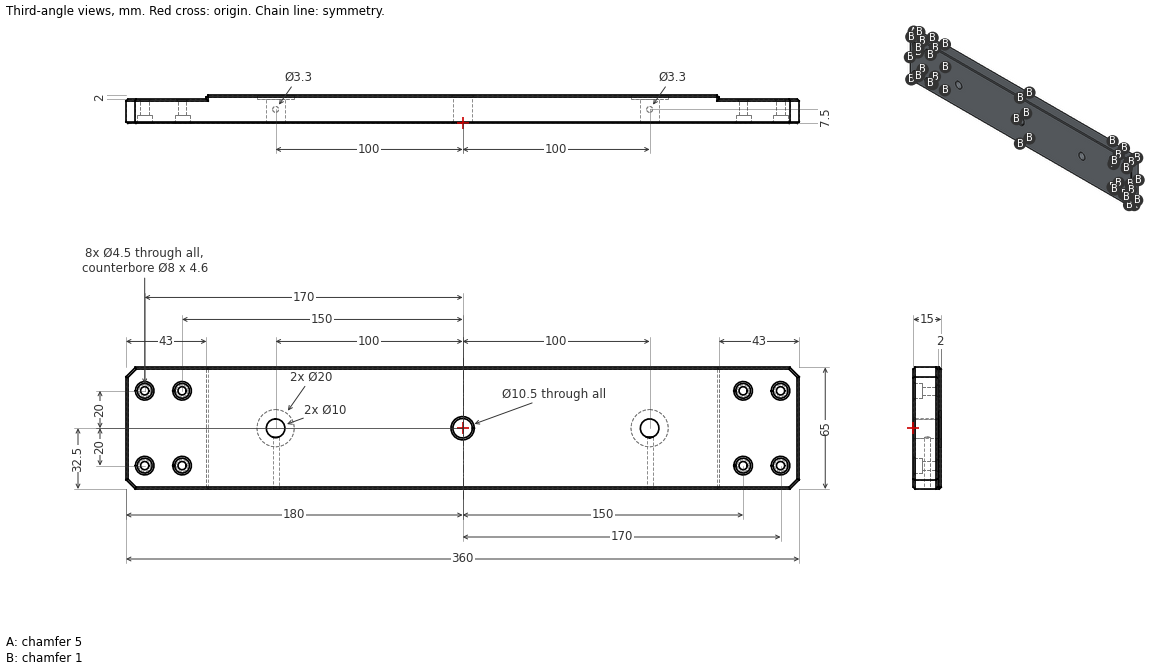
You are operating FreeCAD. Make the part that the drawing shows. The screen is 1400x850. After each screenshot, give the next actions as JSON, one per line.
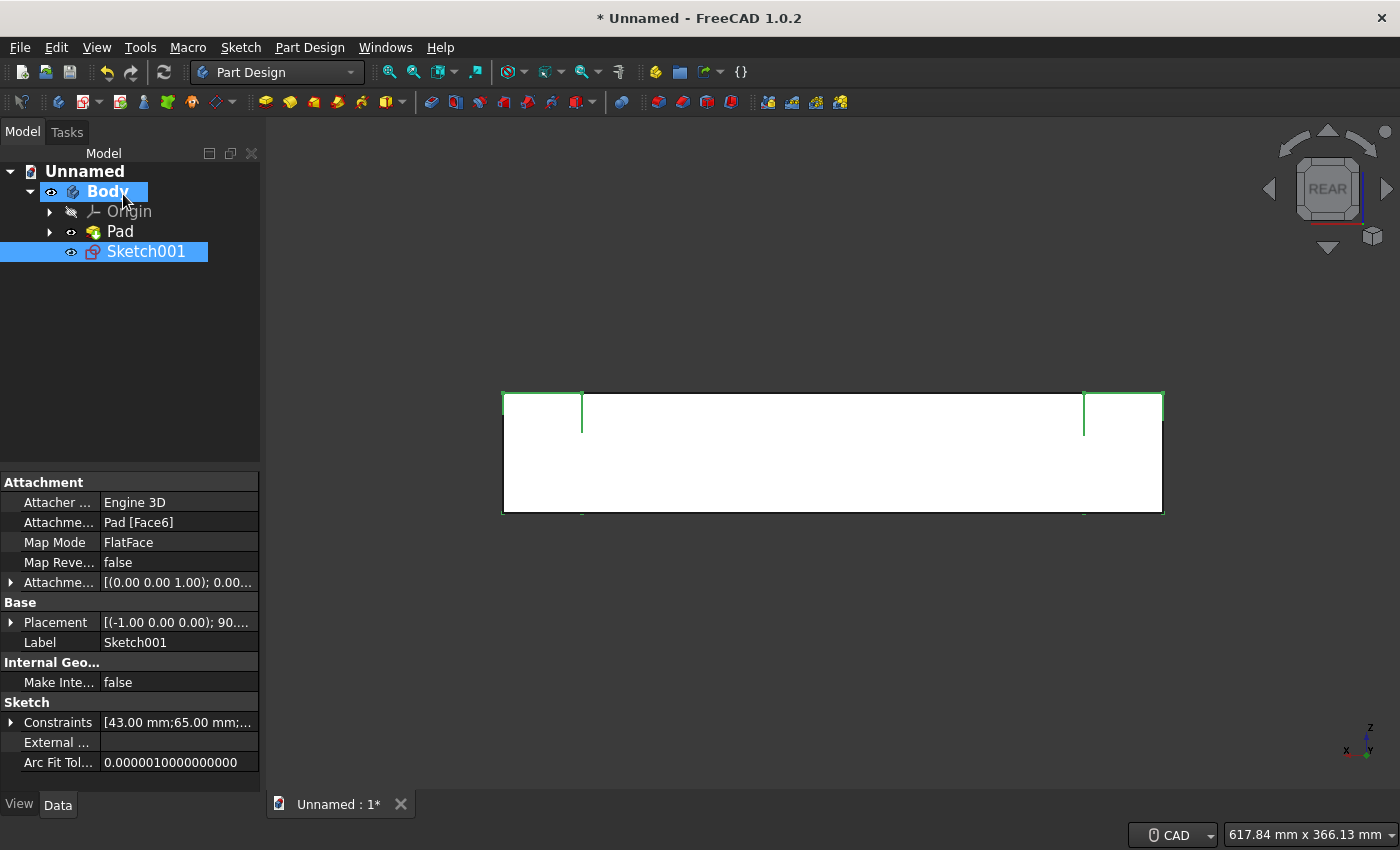
{"action": "left_click", "coordinate": [432, 102]}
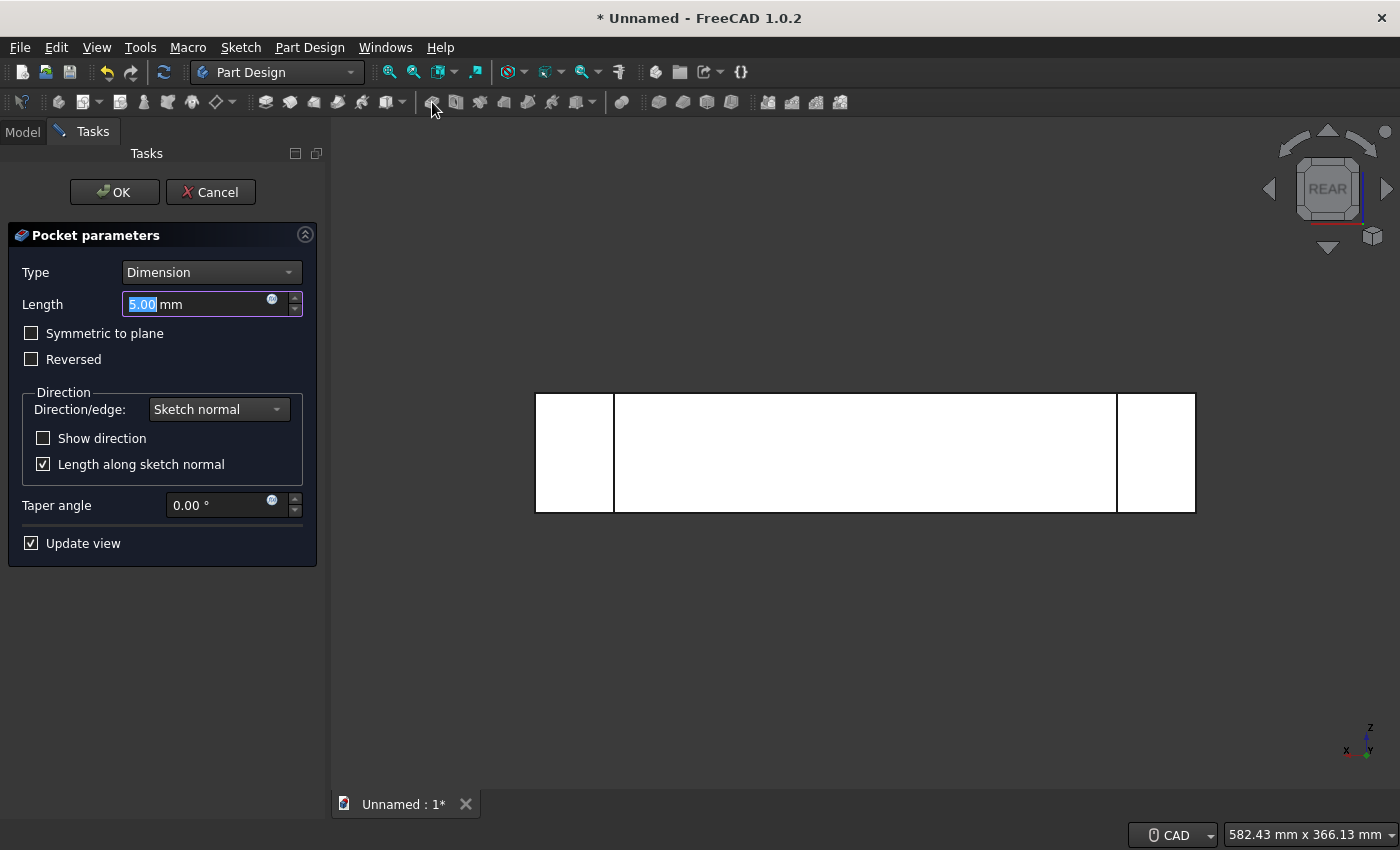
{"action": "type", "text": "2"}
{"action": "key", "text": "Tab"}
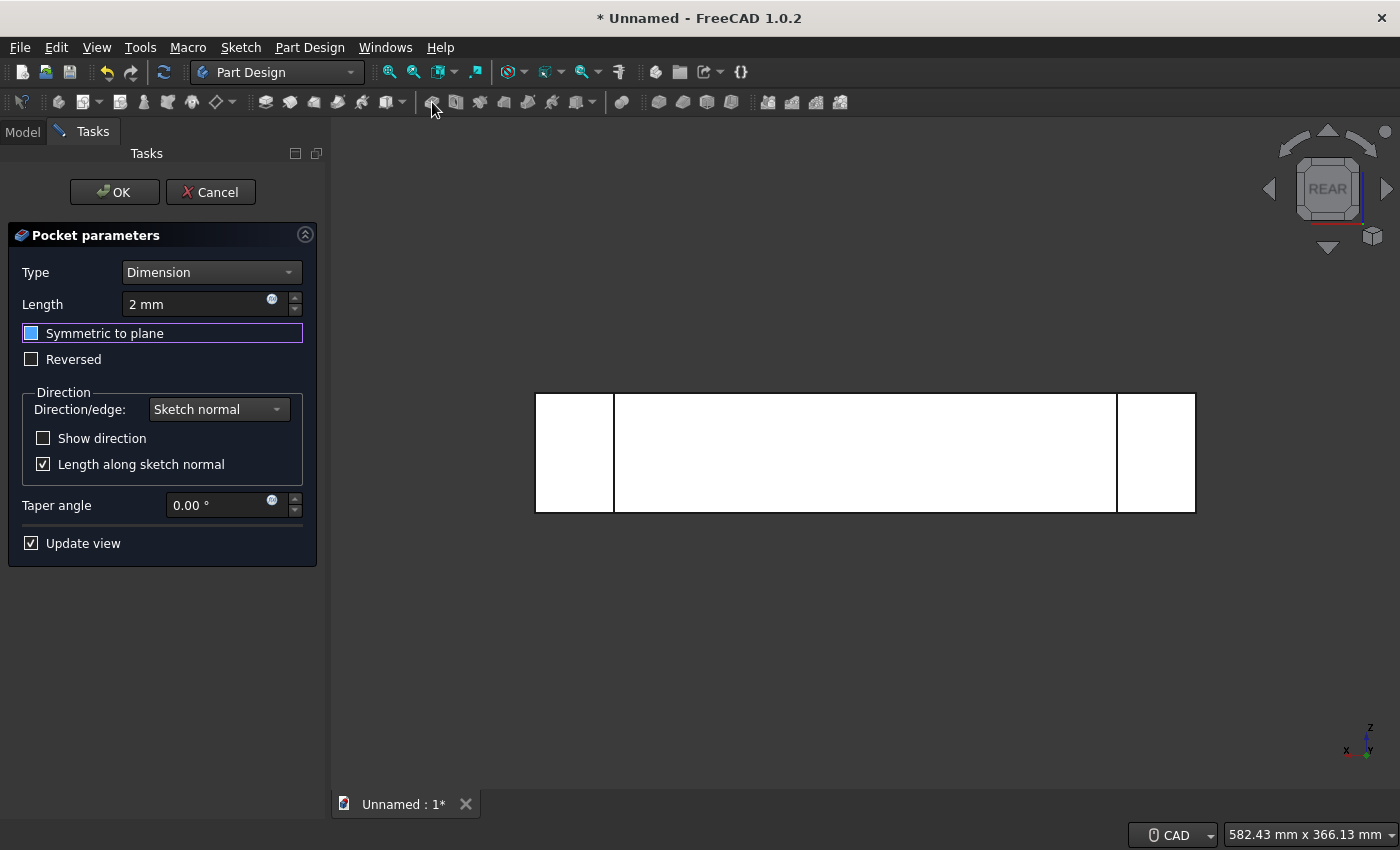
{"action": "left_click", "coordinate": [115, 192]}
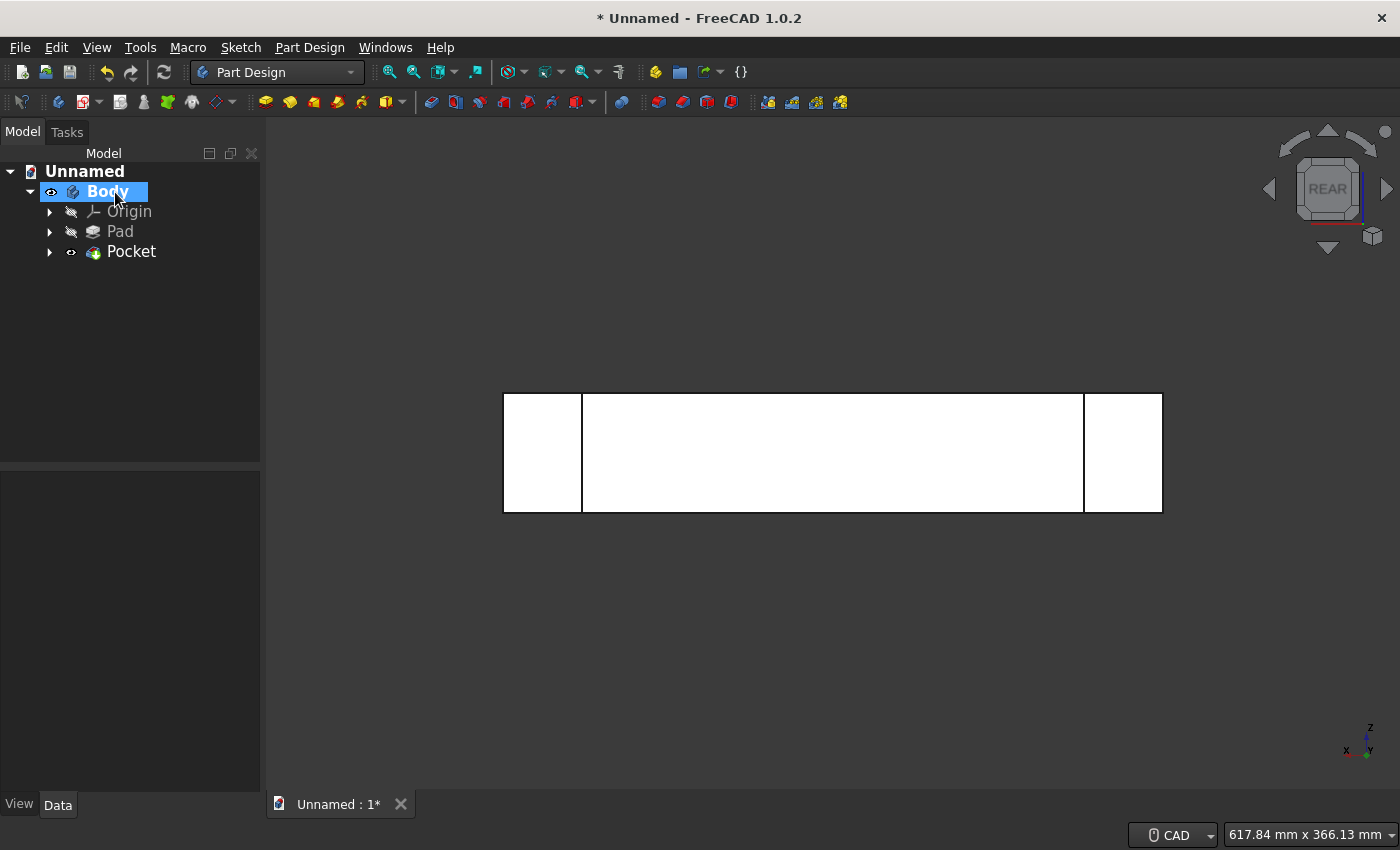
{"action": "left_click", "coordinate": [84, 102]}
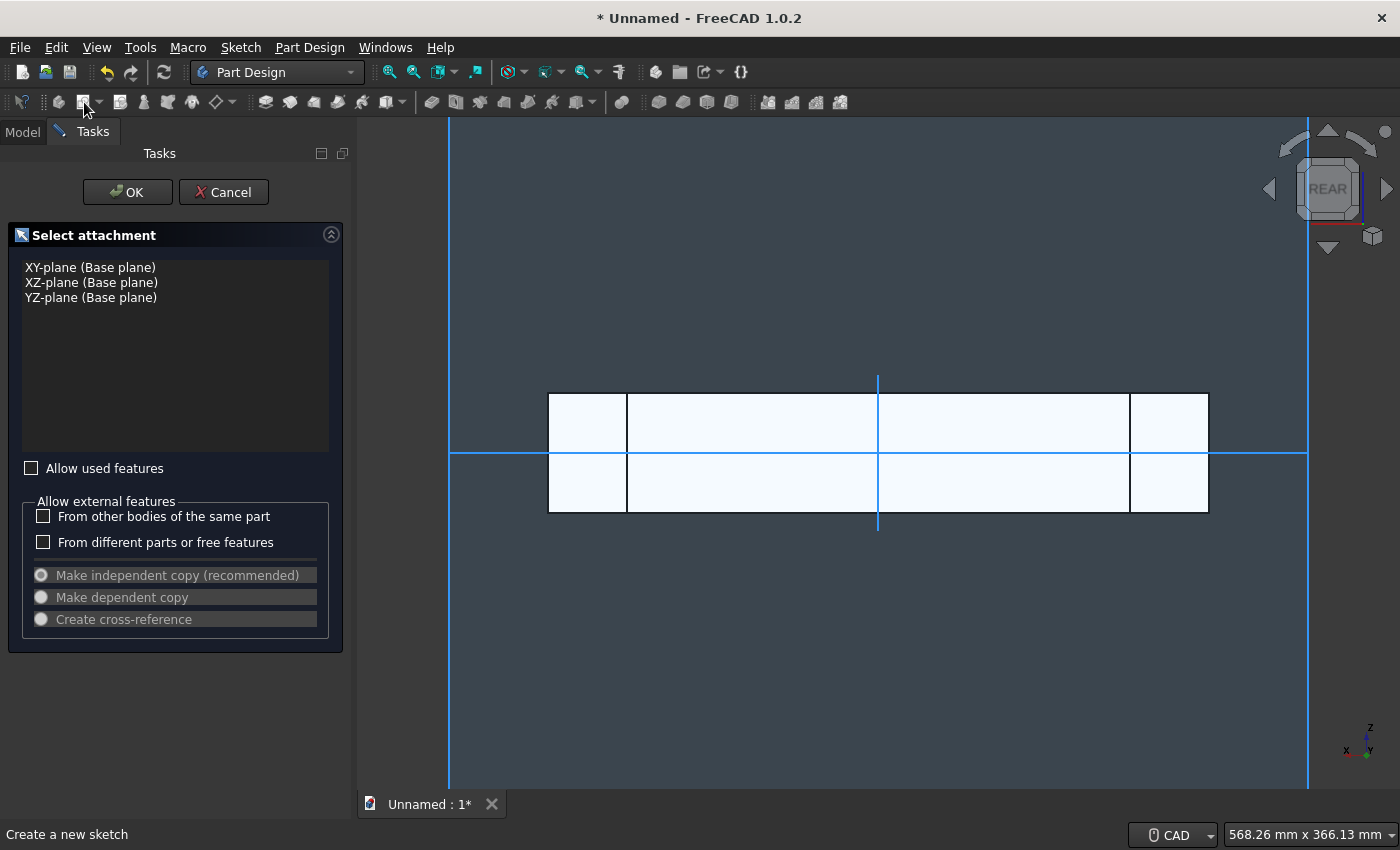
{"action": "left_click", "coordinate": [82, 282]}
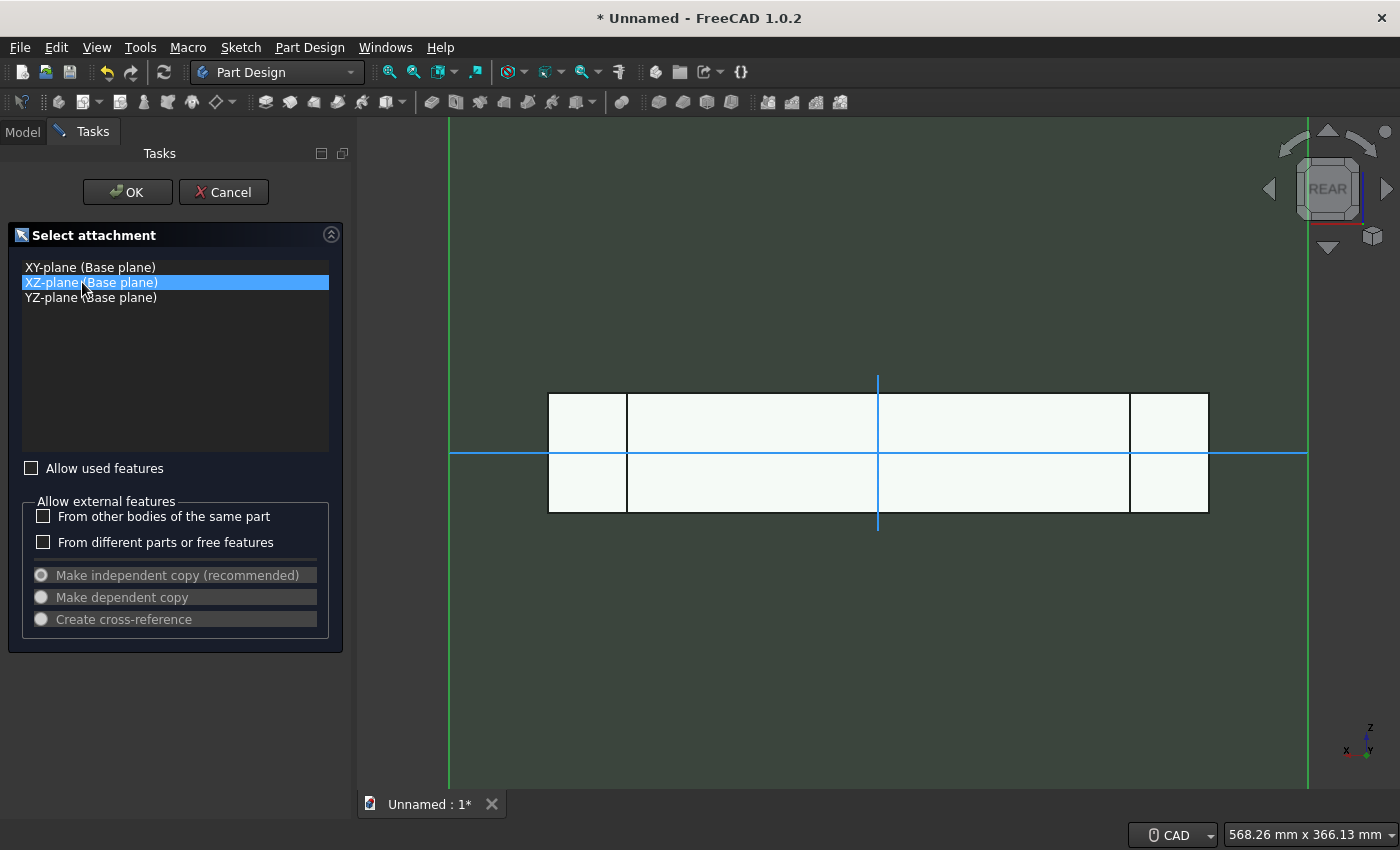
{"action": "left_click", "coordinate": [128, 192]}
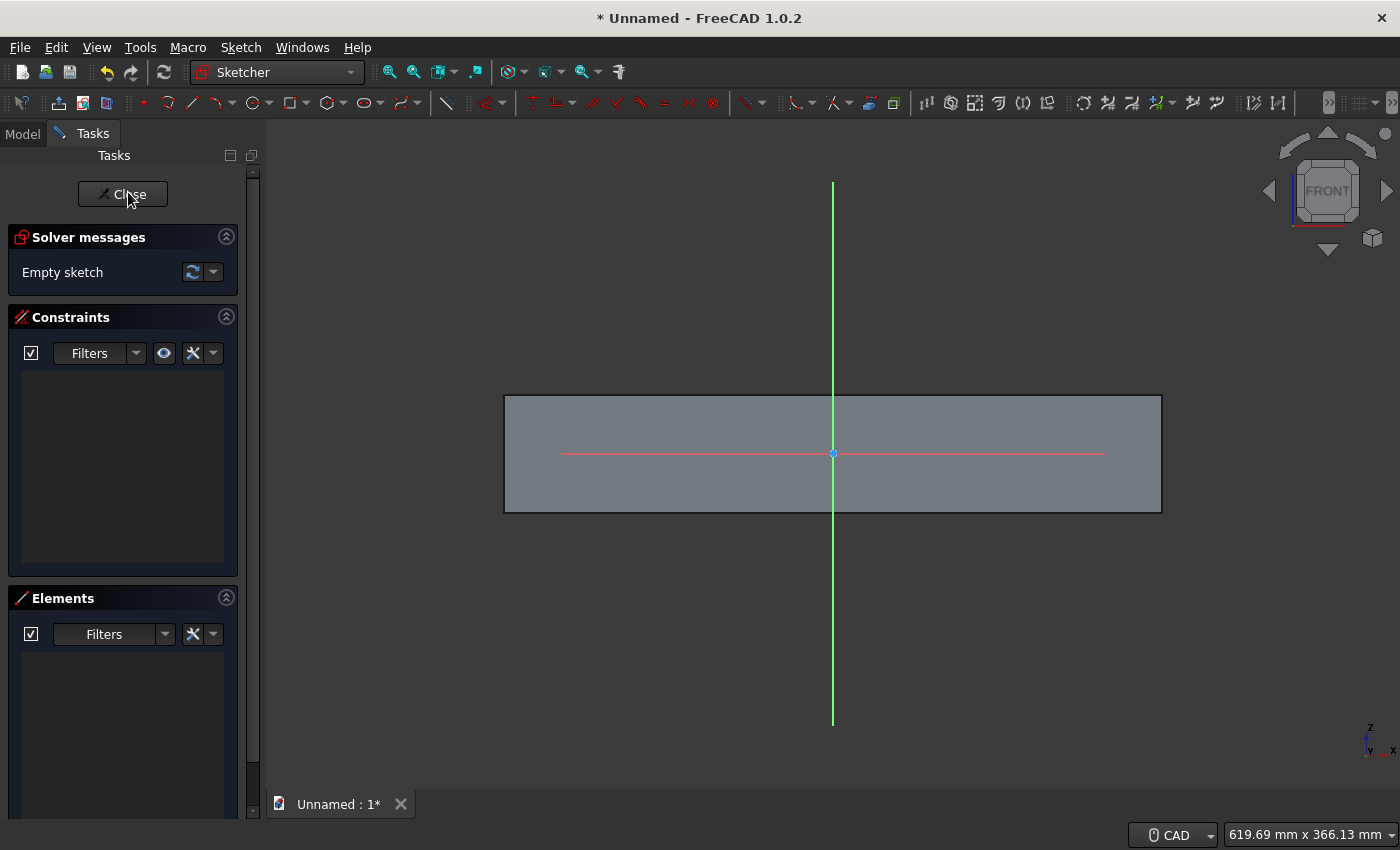
{"action": "left_click", "coordinate": [254, 104]}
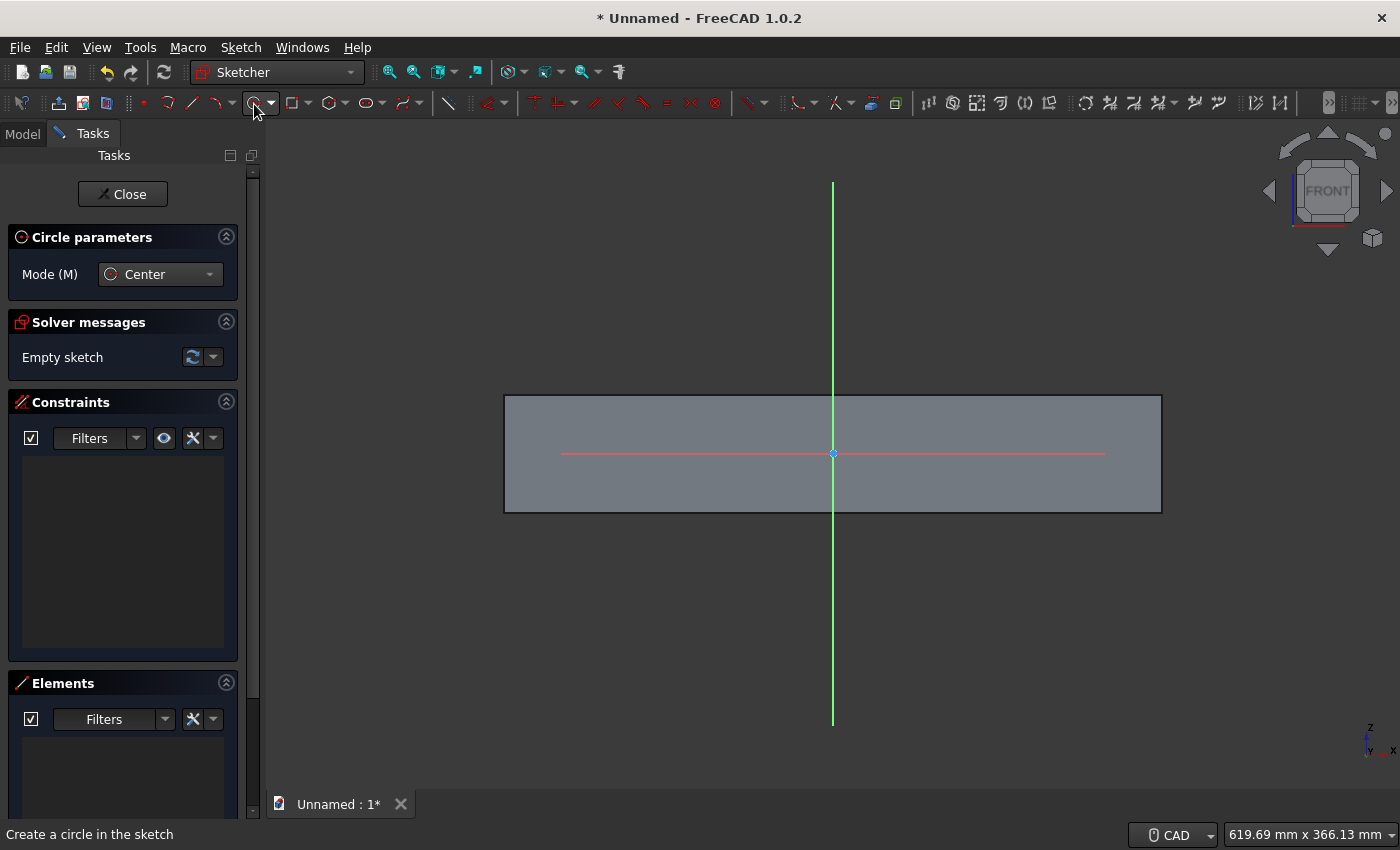
{"action": "scroll", "coordinate": [522, 417], "scroll_direction": "up", "scroll_amount": 9}